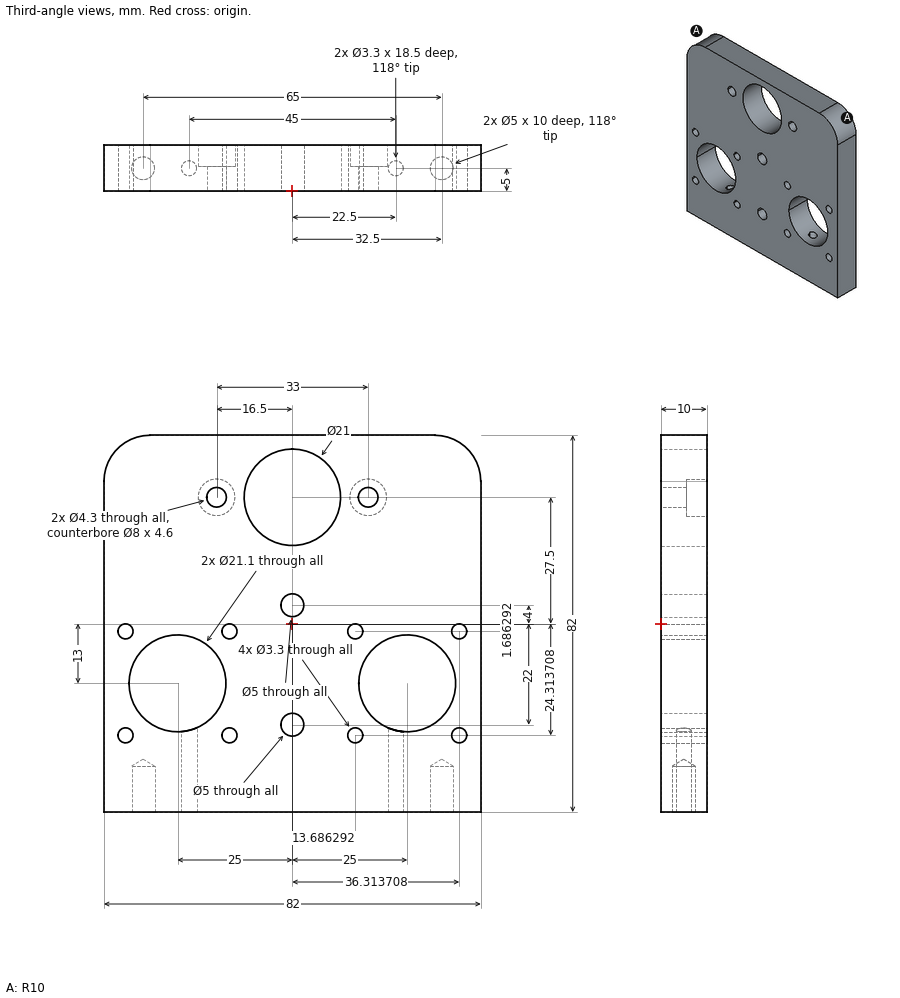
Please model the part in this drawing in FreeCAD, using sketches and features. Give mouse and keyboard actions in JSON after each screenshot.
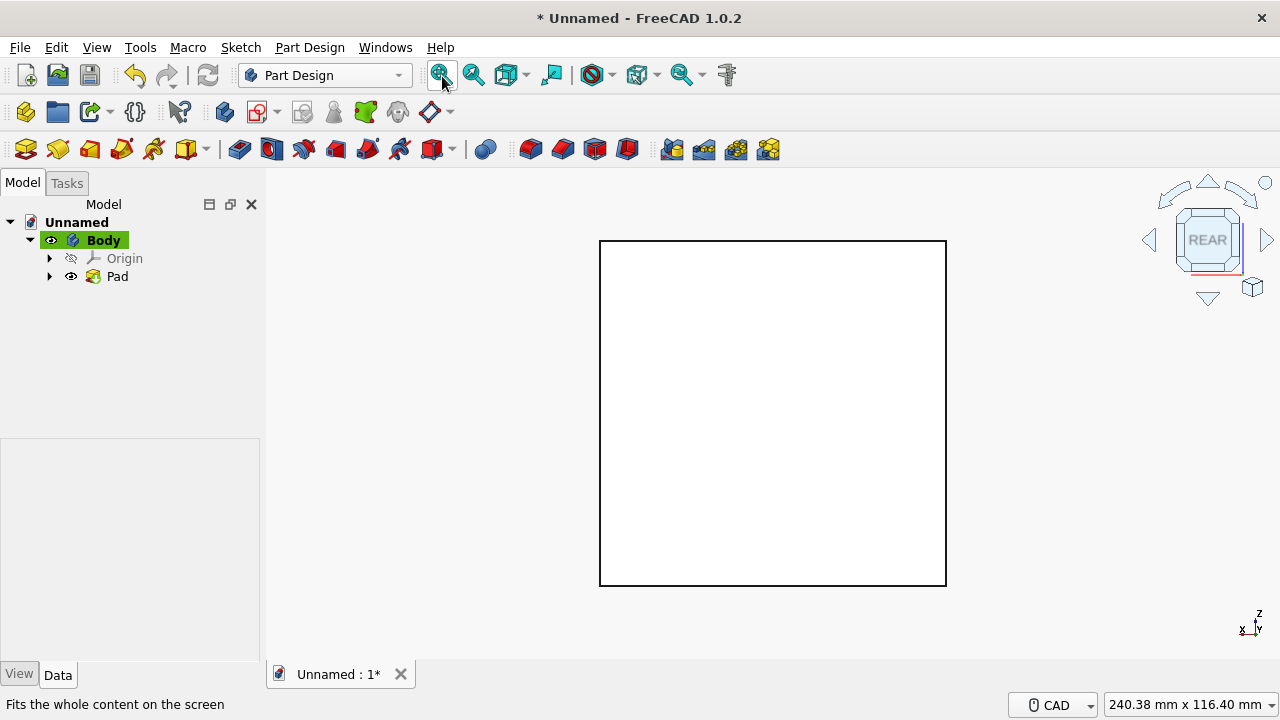
{"action": "left_click", "coordinate": [773, 413]}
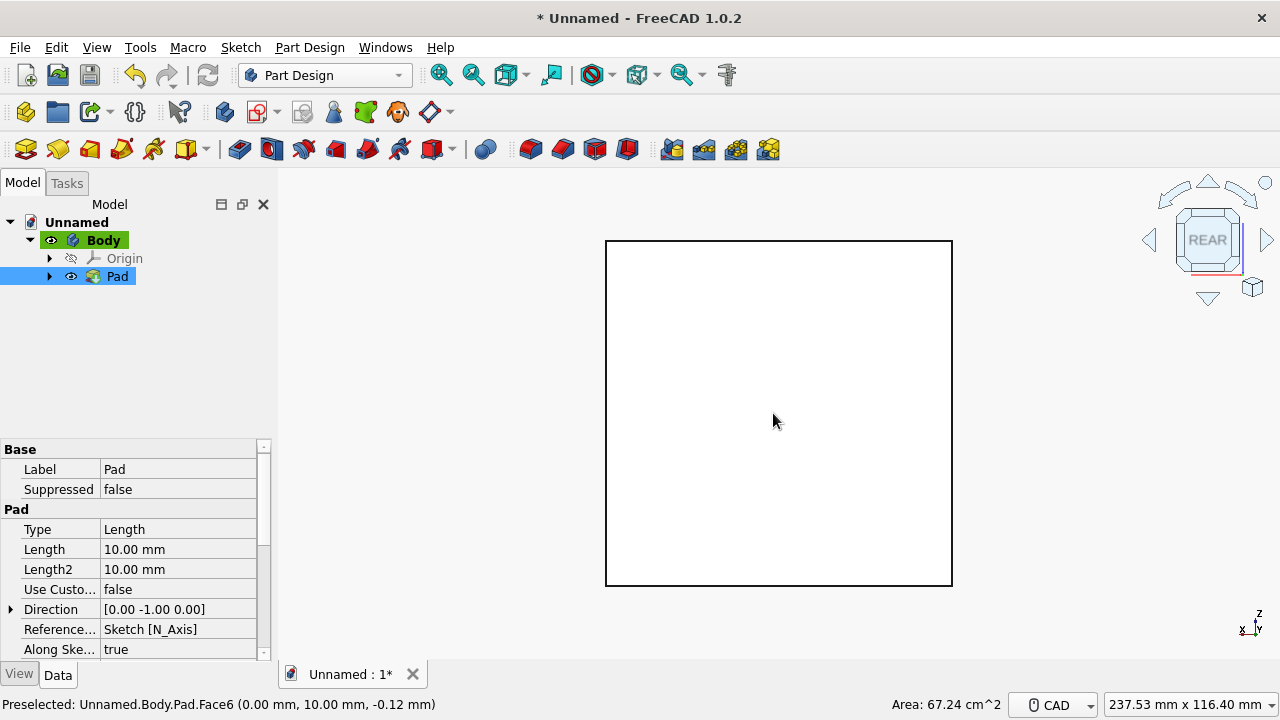
{"action": "left_click", "coordinate": [258, 112]}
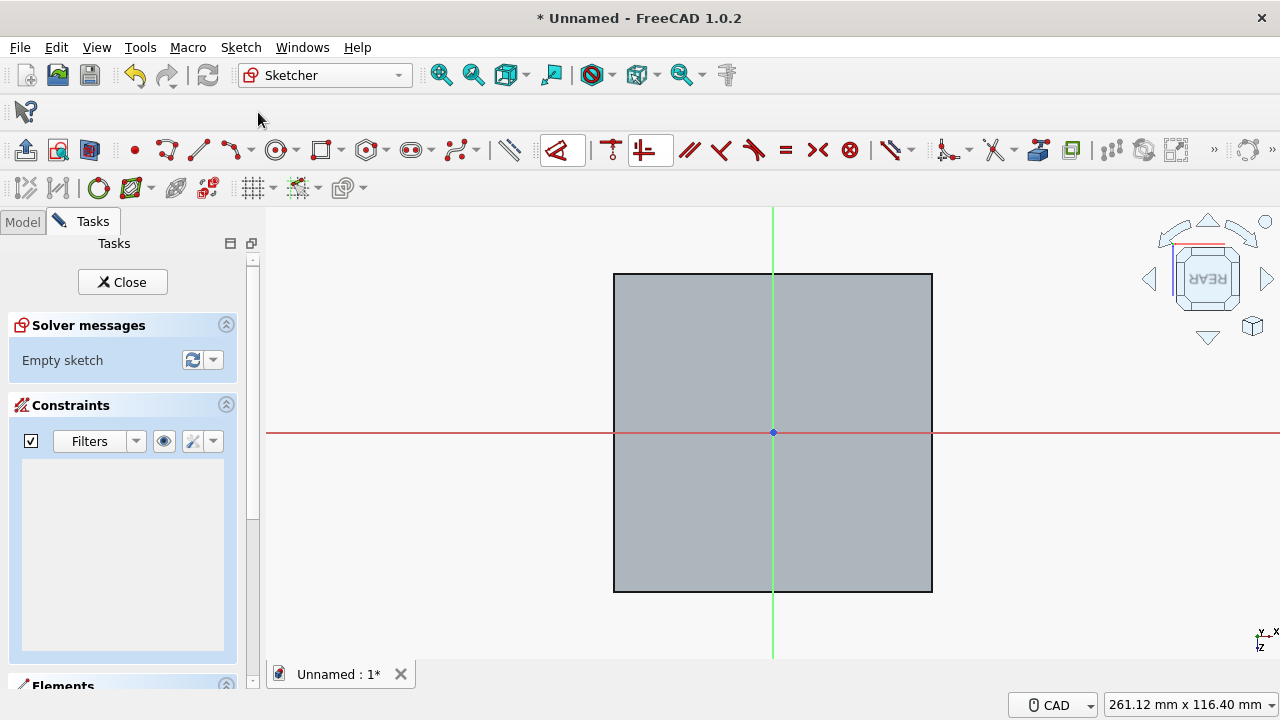
{"action": "scroll", "coordinate": [856, 597], "scroll_direction": "up", "scroll_amount": 3}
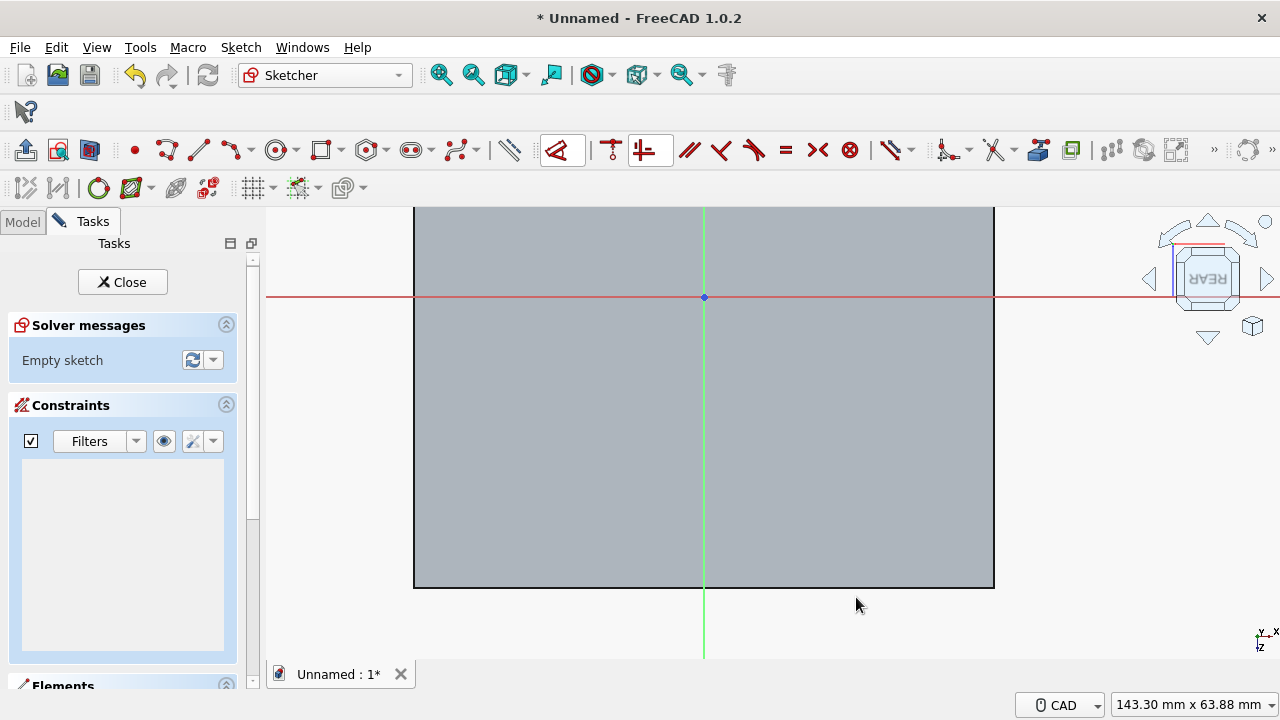
{"action": "left_click", "coordinate": [276, 150]}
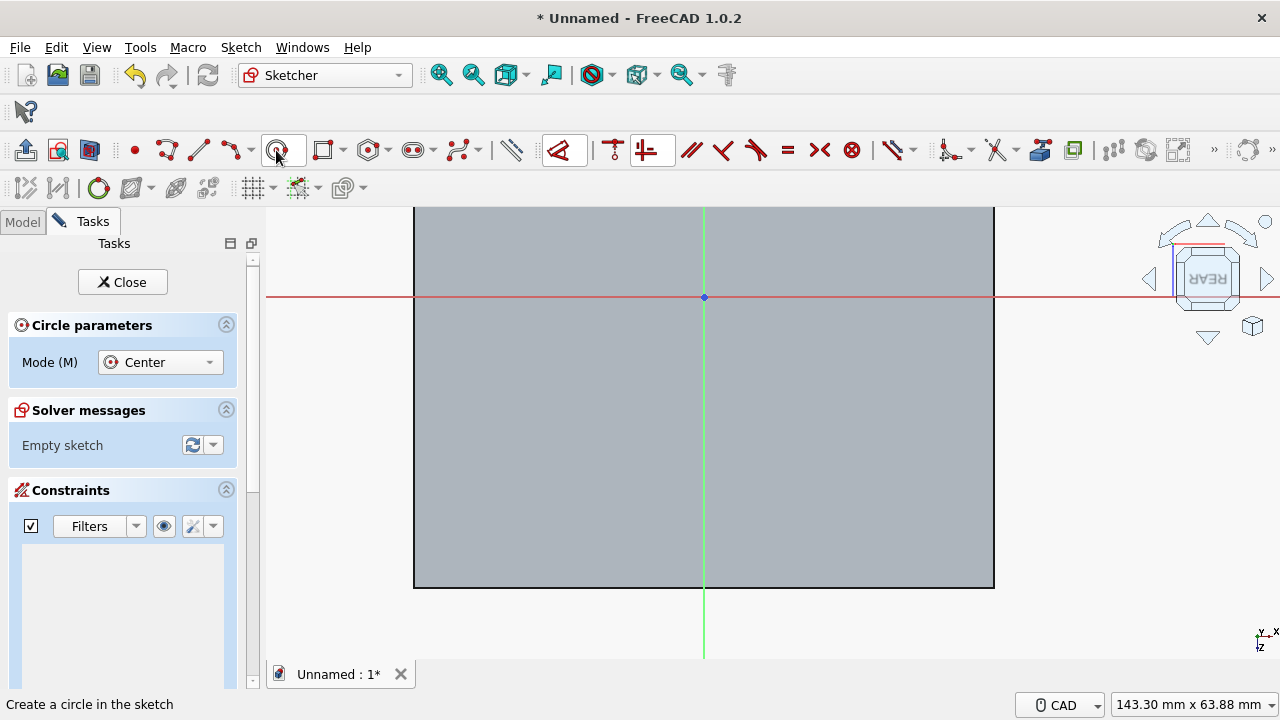
{"action": "left_click", "coordinate": [704, 492]}
{"action": "left_click", "coordinate": [757, 440]}
{"action": "key", "text": "Escape"}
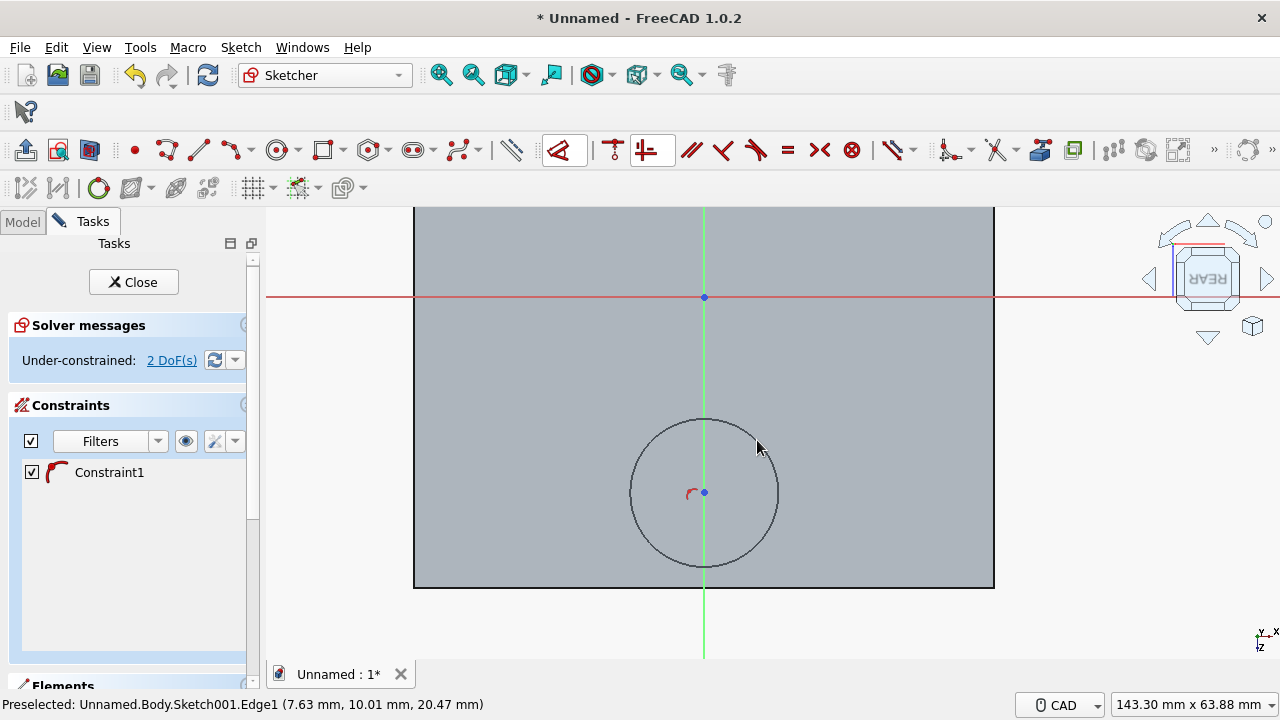
{"action": "left_click", "coordinate": [756, 440]}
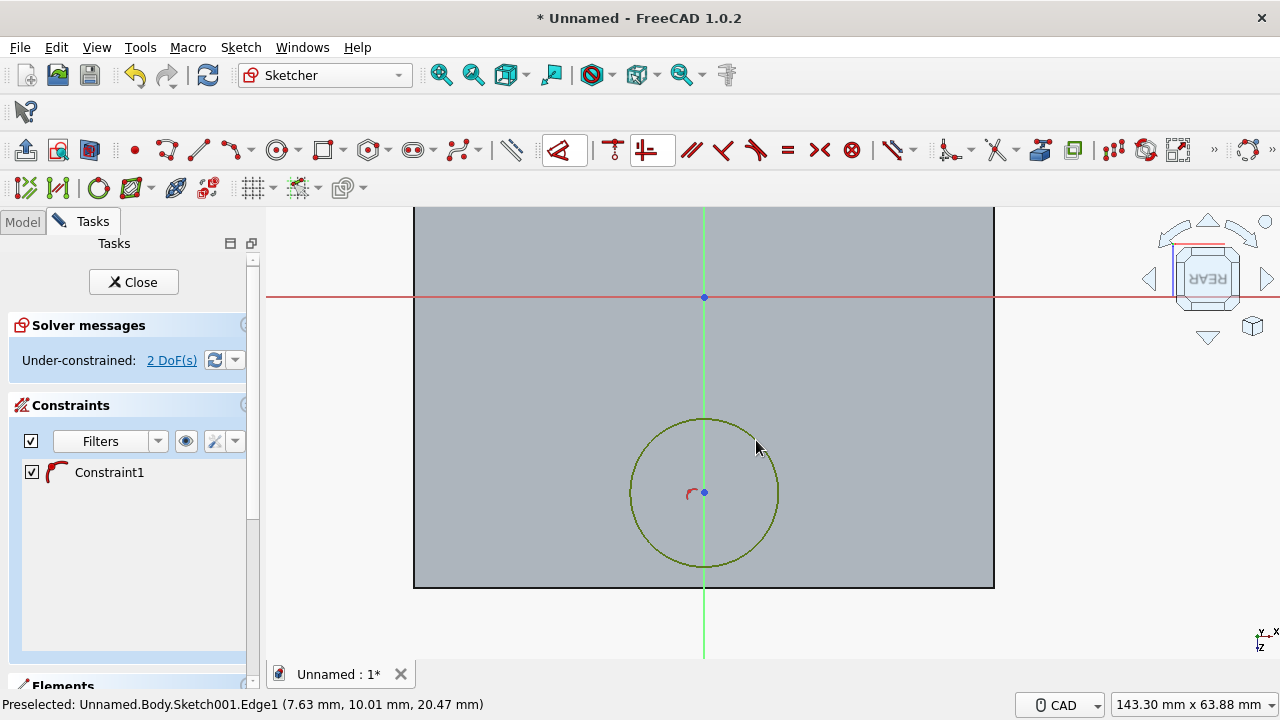
{"action": "left_click", "coordinate": [582, 150]}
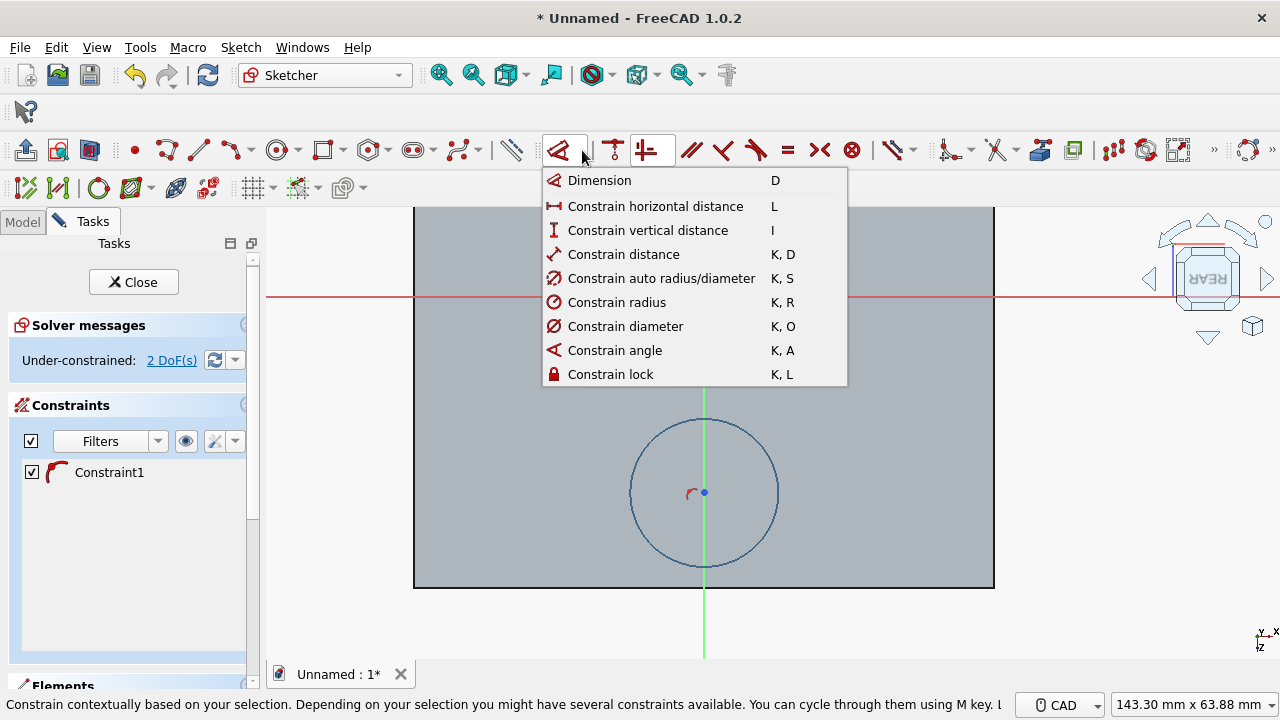
{"action": "left_click", "coordinate": [695, 326]}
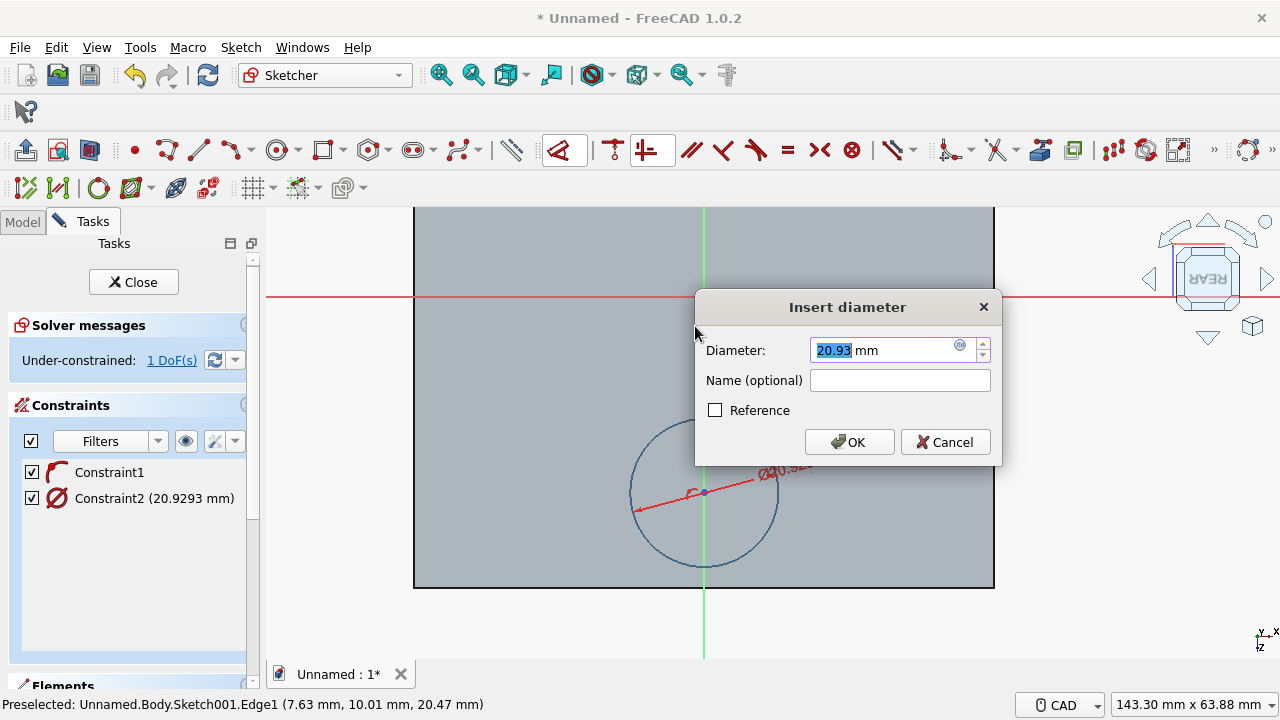
{"action": "type", "text": "21"}
{"action": "key", "text": "Return"}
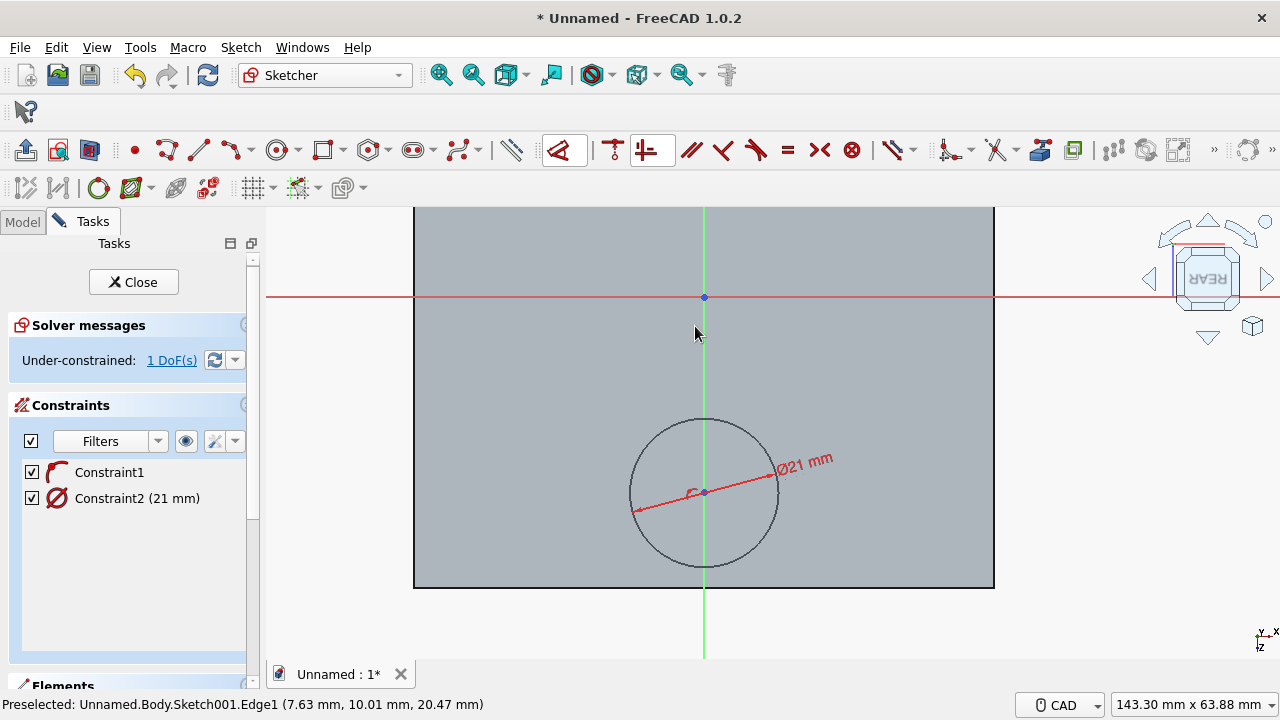
{"action": "left_click", "coordinate": [704, 493]}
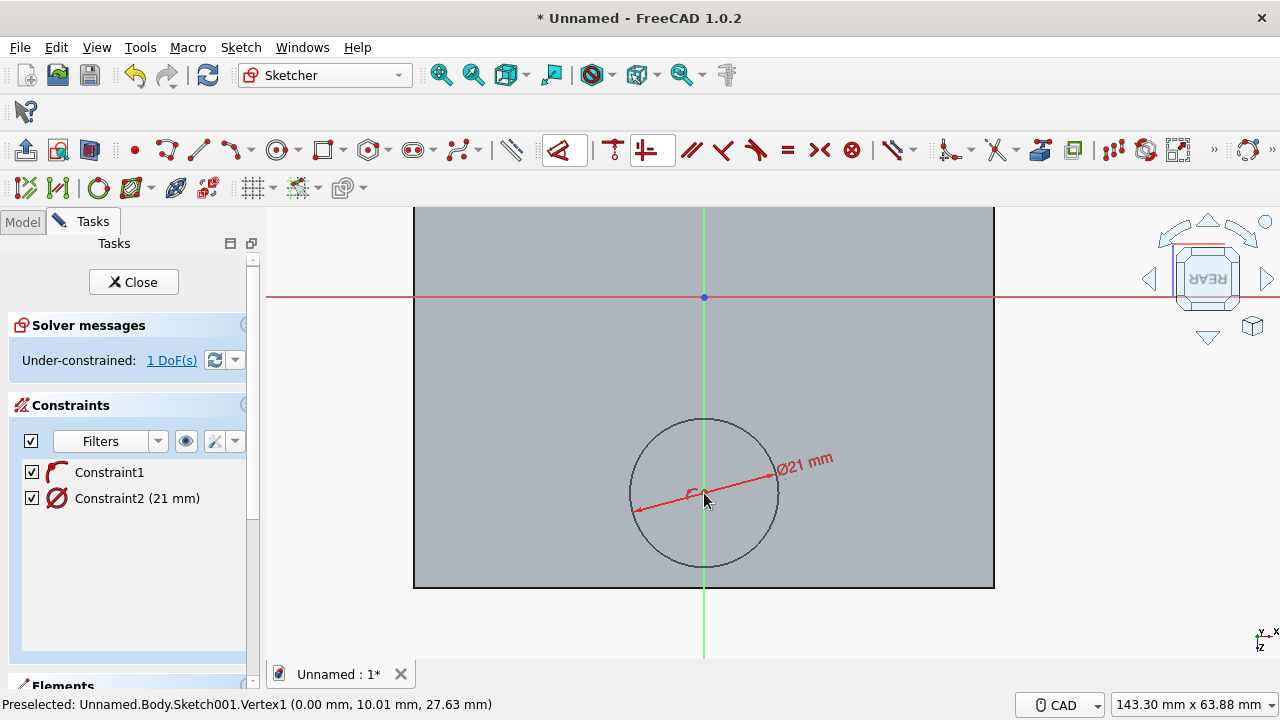
{"action": "left_click", "coordinate": [582, 150]}